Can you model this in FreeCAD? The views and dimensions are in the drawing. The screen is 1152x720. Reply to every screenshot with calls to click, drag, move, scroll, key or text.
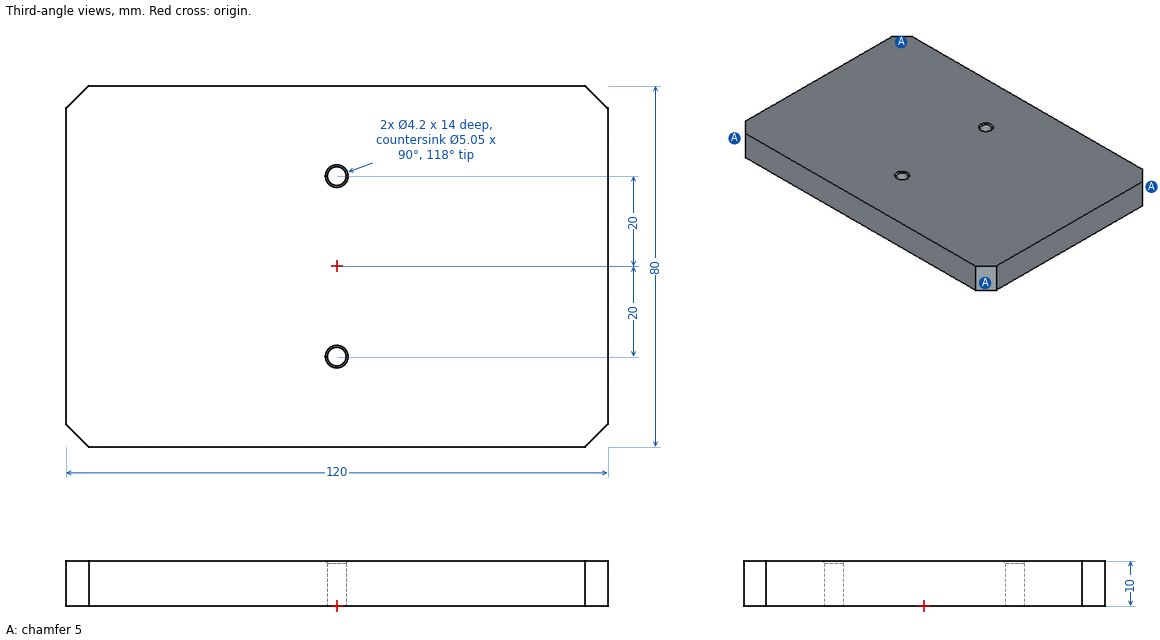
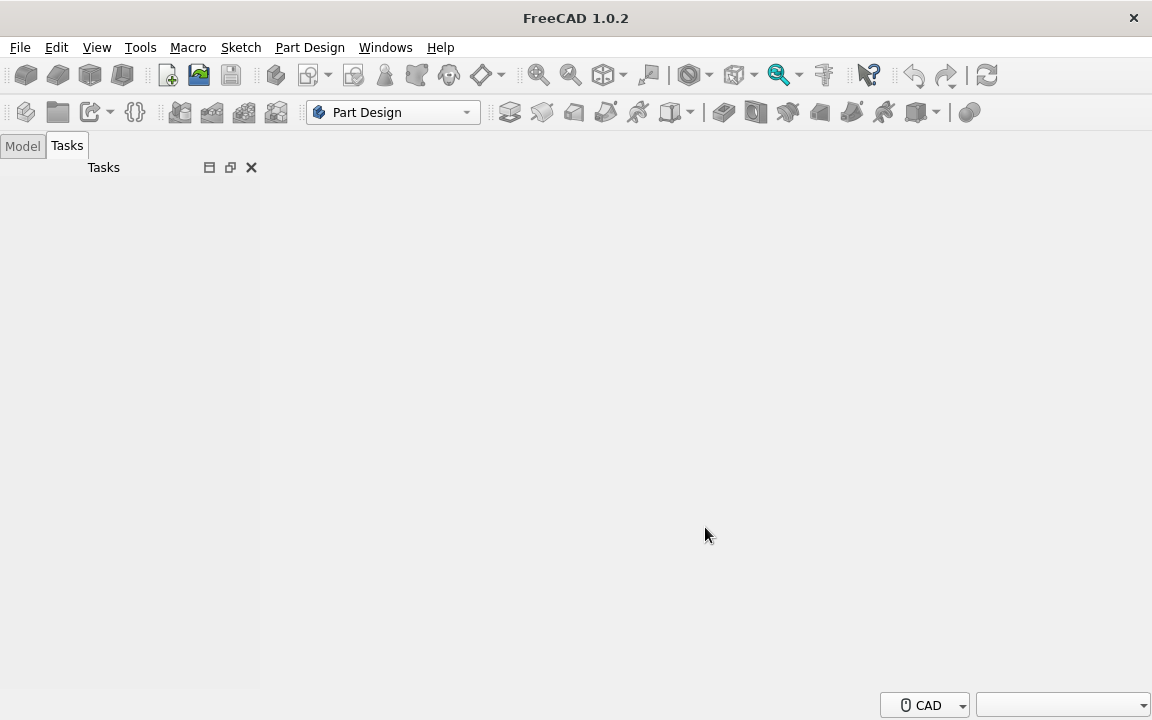
key(ctrl+n)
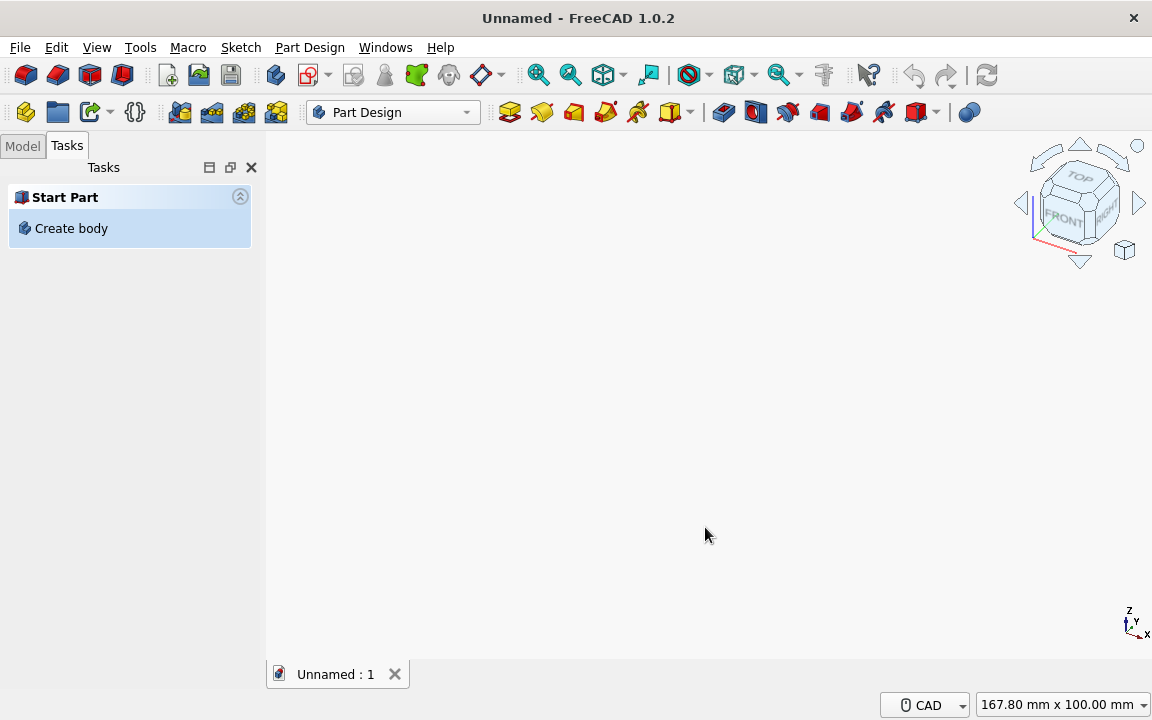
click(308, 76)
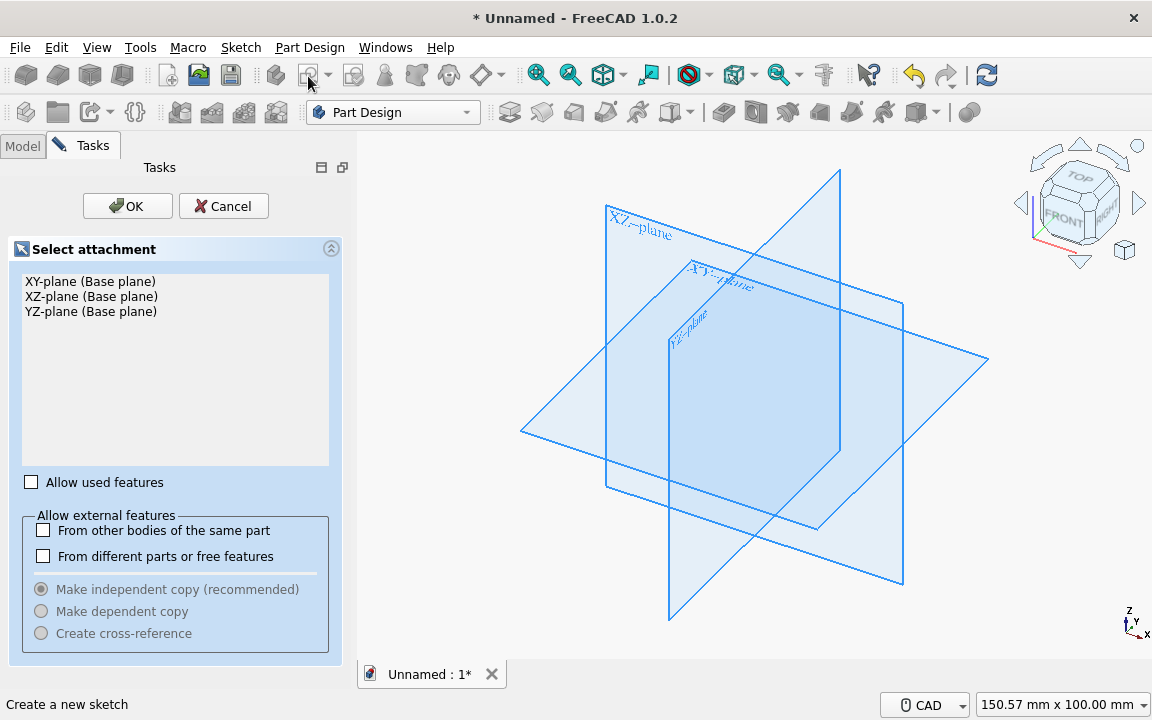
click(82, 282)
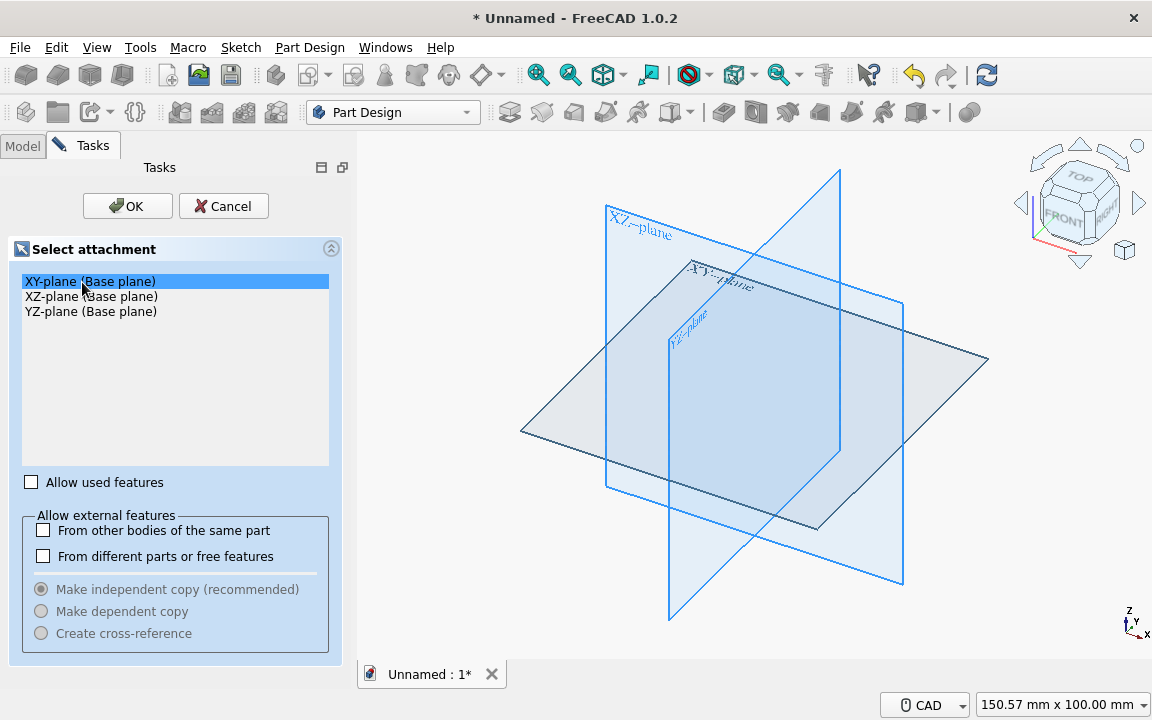
click(128, 206)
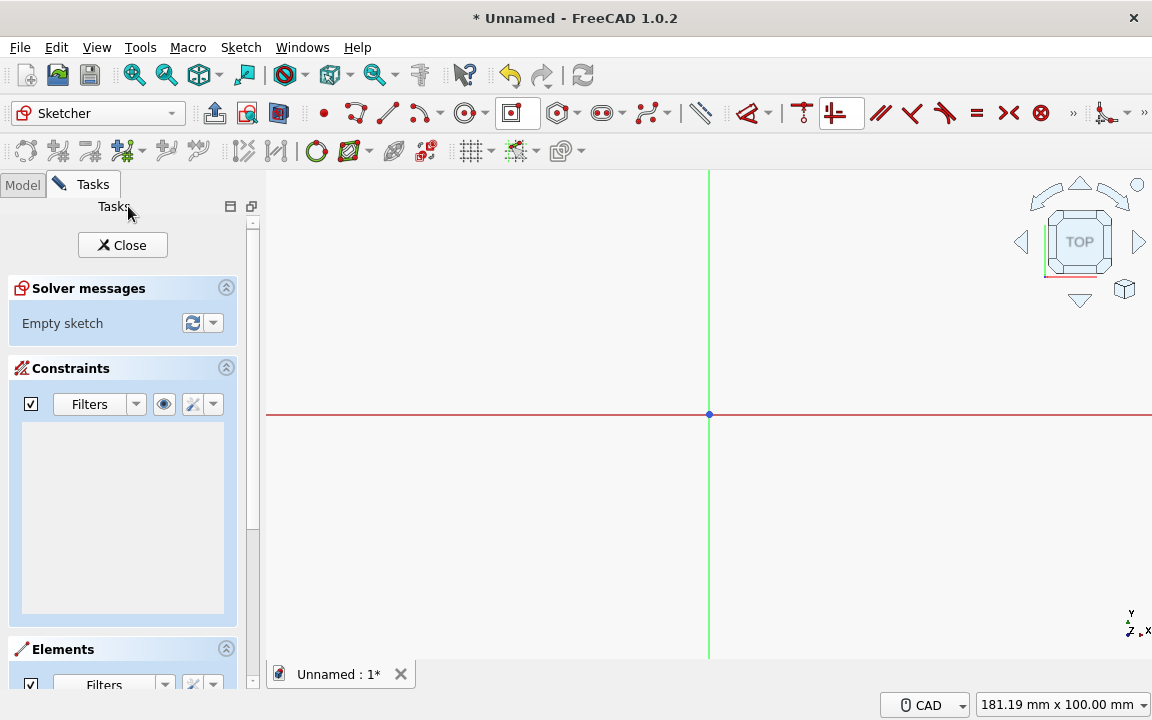
scroll(331, 415, down, 1)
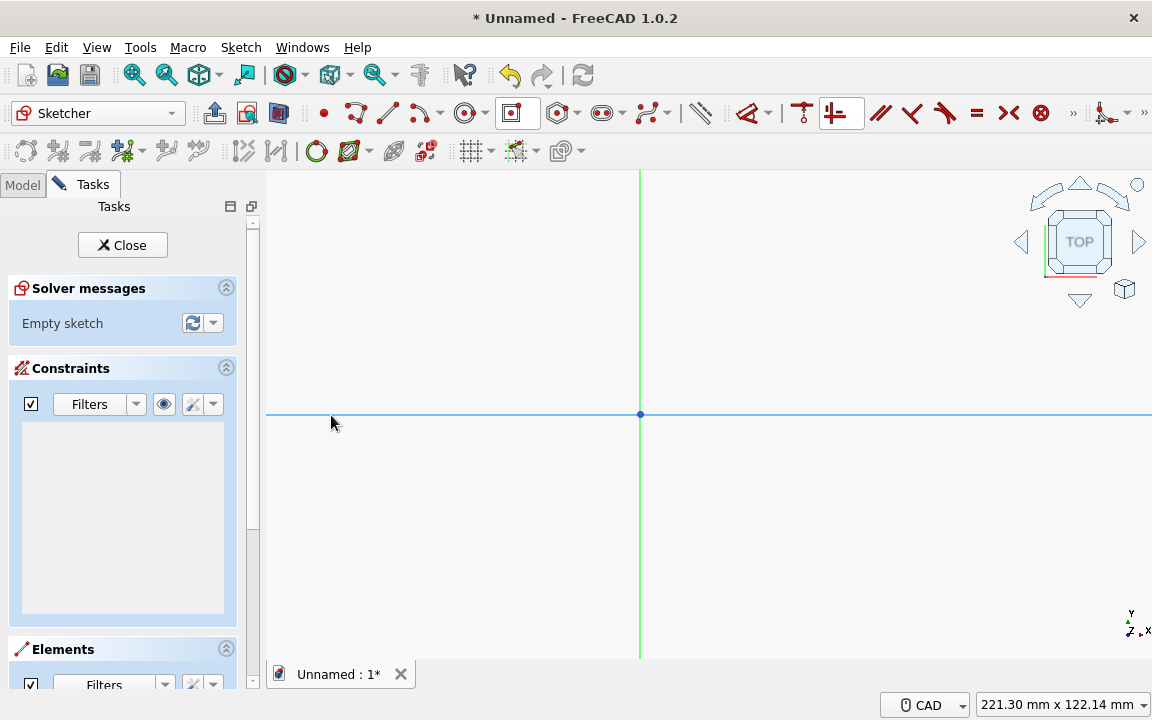
key(g)
key(v)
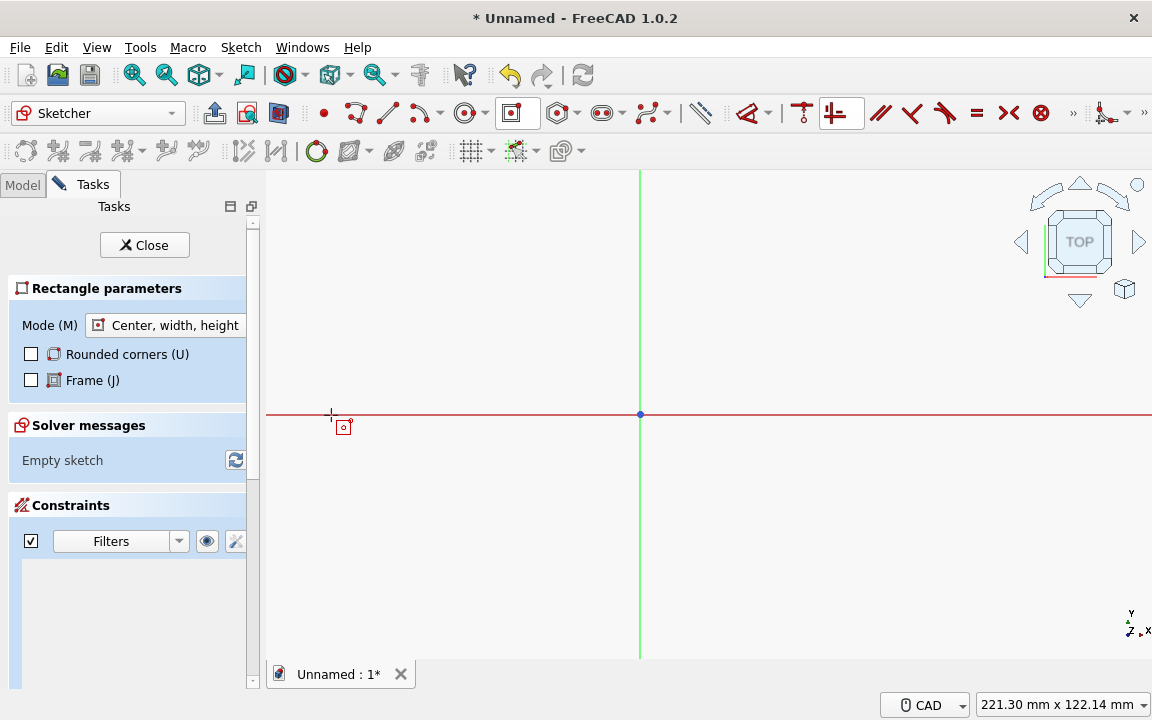
click(640, 415)
click(881, 255)
key(Escape)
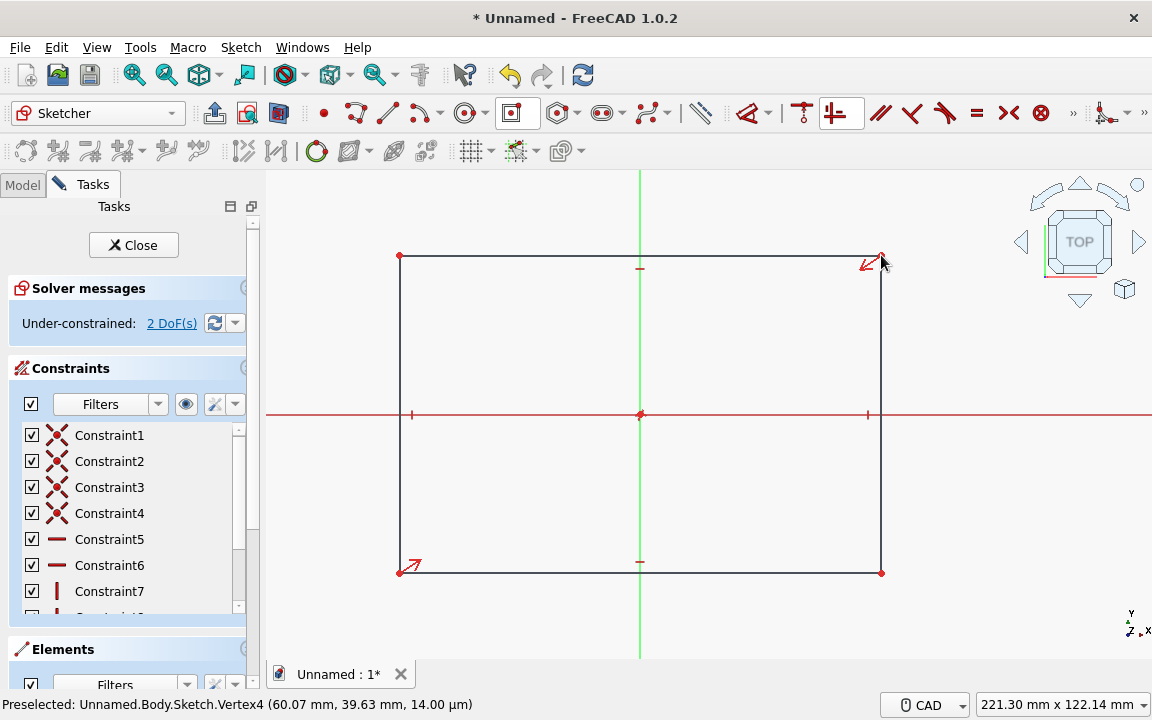
key(d)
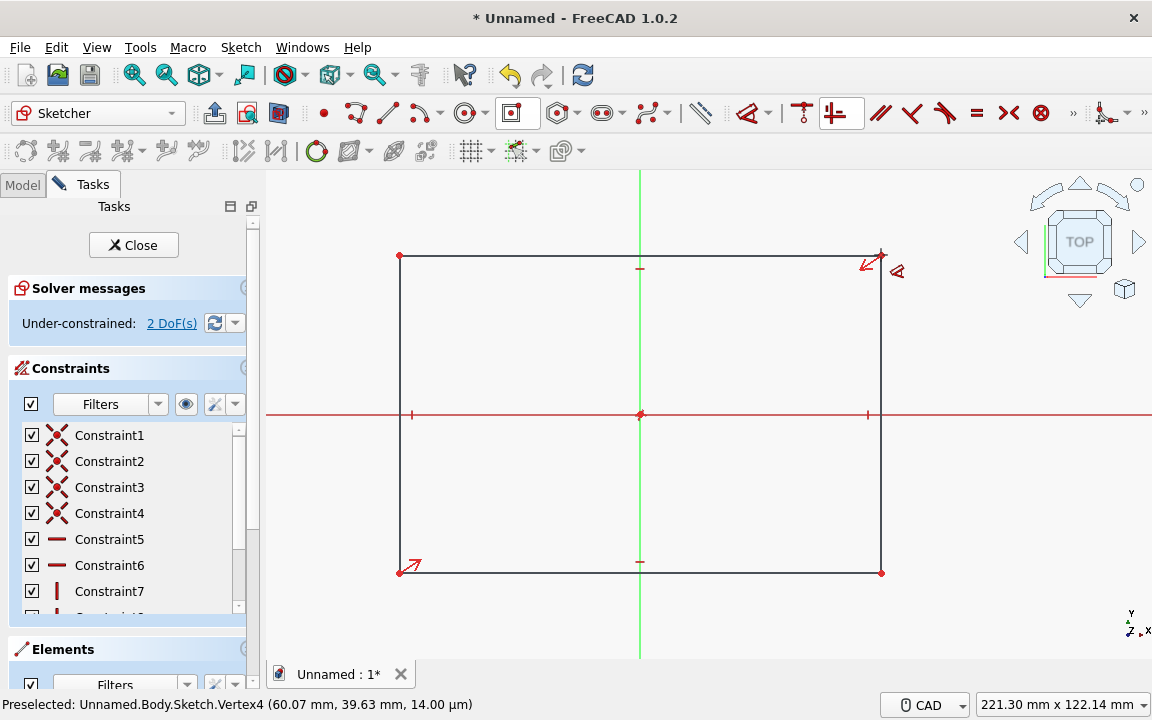
click(881, 478)
click(915, 342)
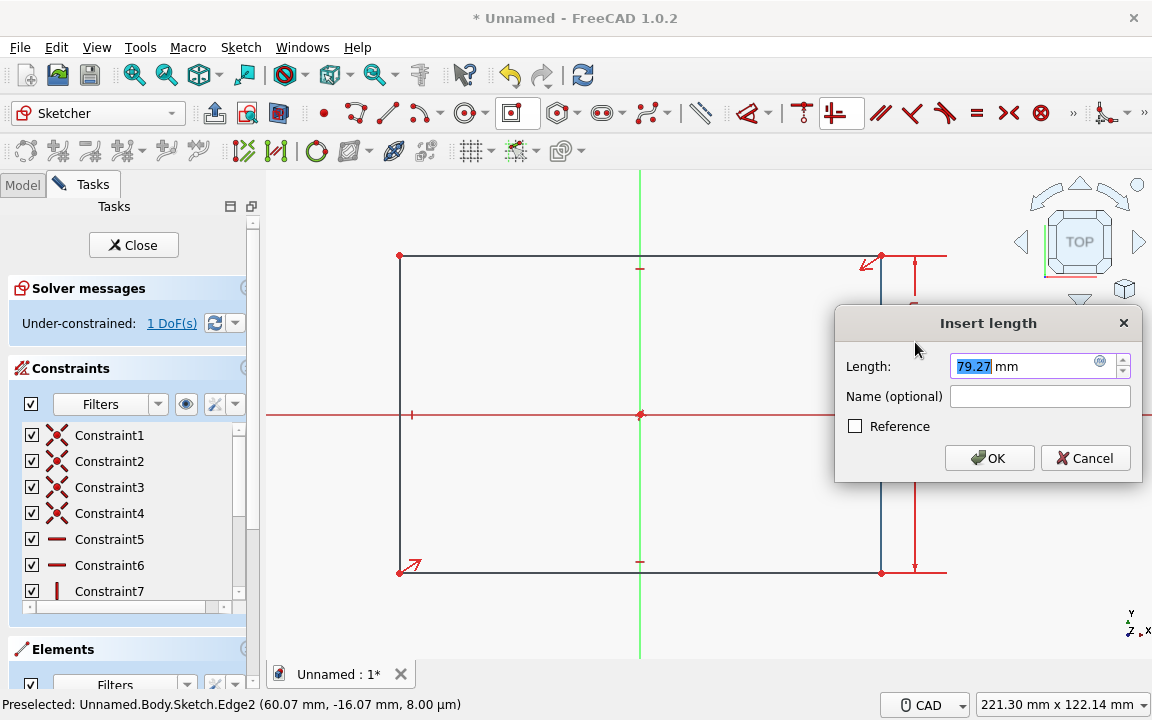
text(80)
key(Return)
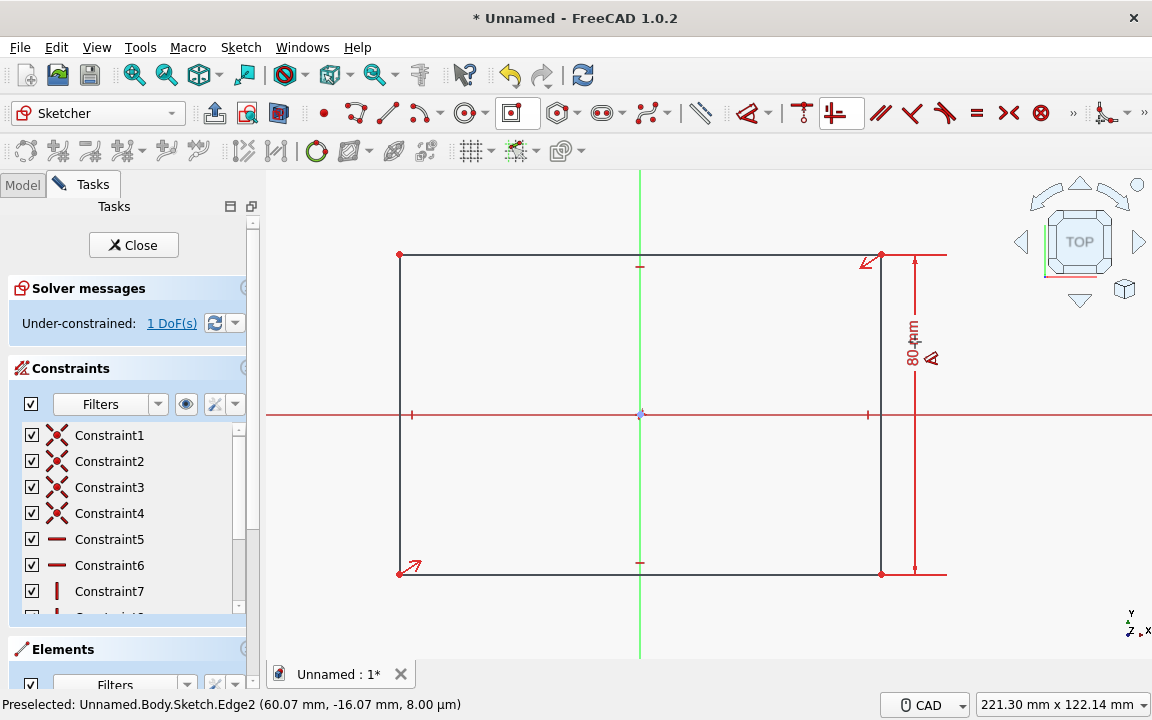
click(544, 575)
click(530, 609)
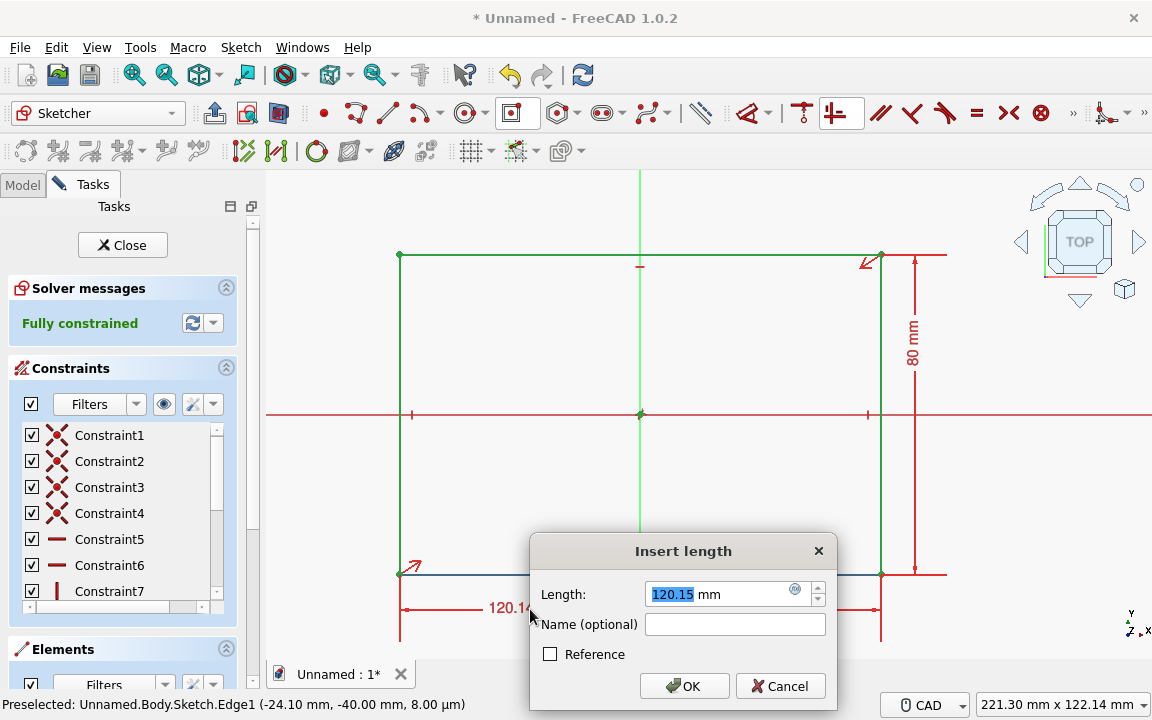
text(120)
key(Return)
key(Escape)